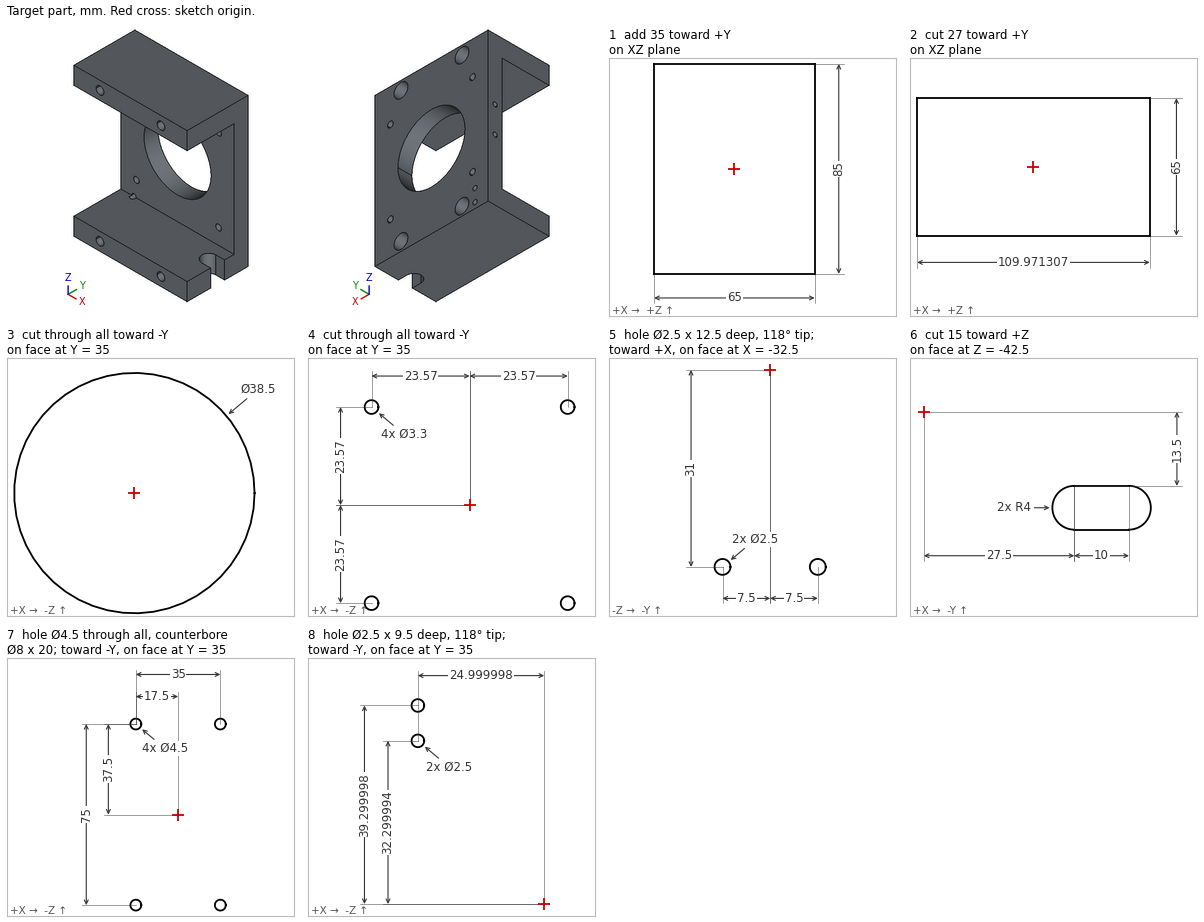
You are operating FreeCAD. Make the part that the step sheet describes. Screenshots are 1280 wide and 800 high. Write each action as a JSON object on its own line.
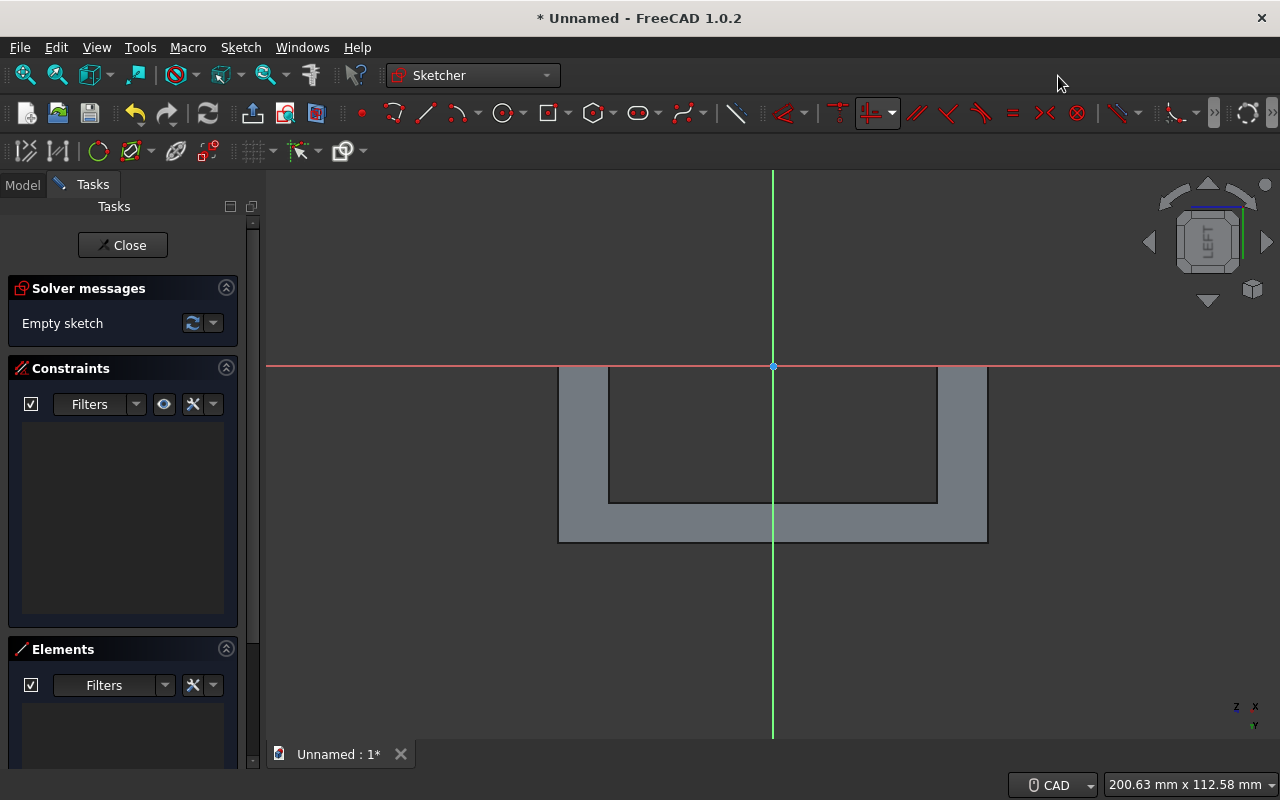
{"action": "scroll", "coordinate": [829, 442], "scroll_direction": "up", "scroll_amount": 4}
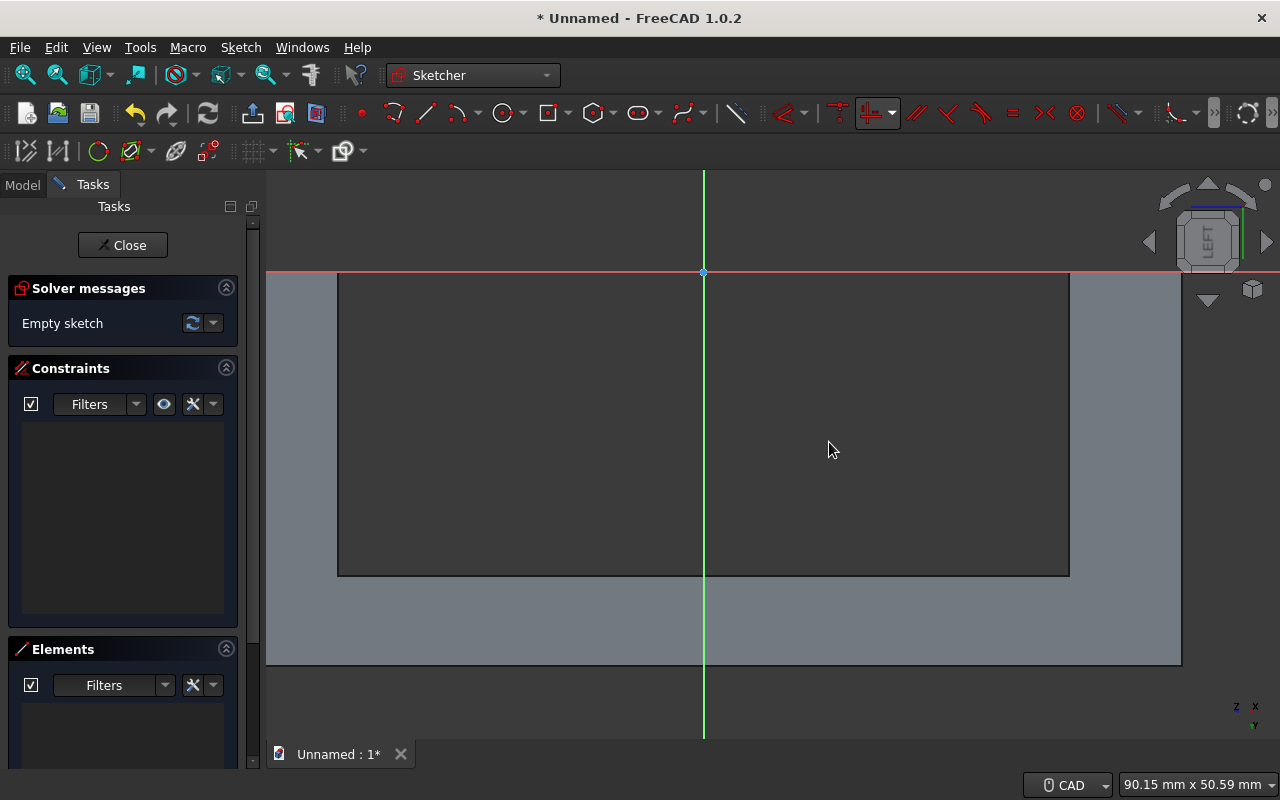
{"action": "left_click", "coordinate": [504, 114]}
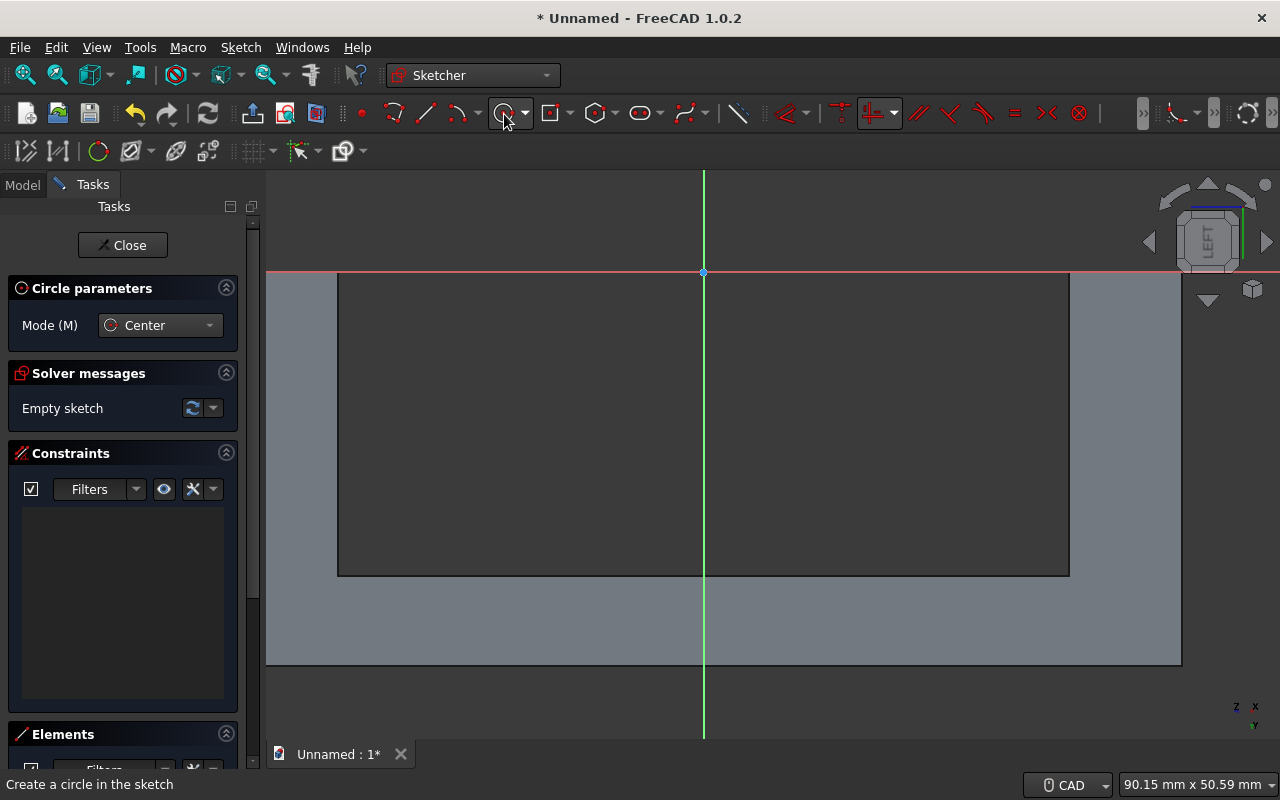
{"action": "scroll", "coordinate": [619, 621], "scroll_direction": "up", "scroll_amount": 3}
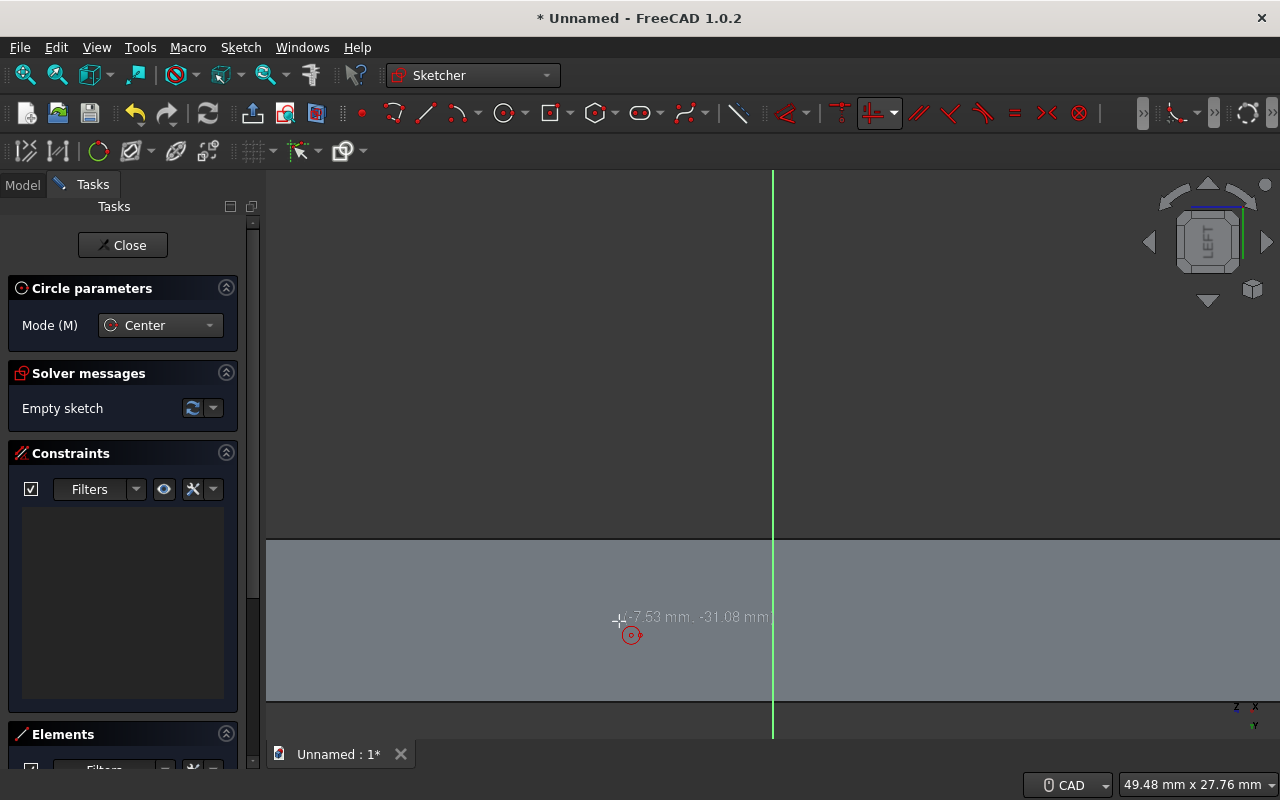
{"action": "left_click", "coordinate": [619, 620]}
{"action": "mouse_move", "coordinate": [637, 602]}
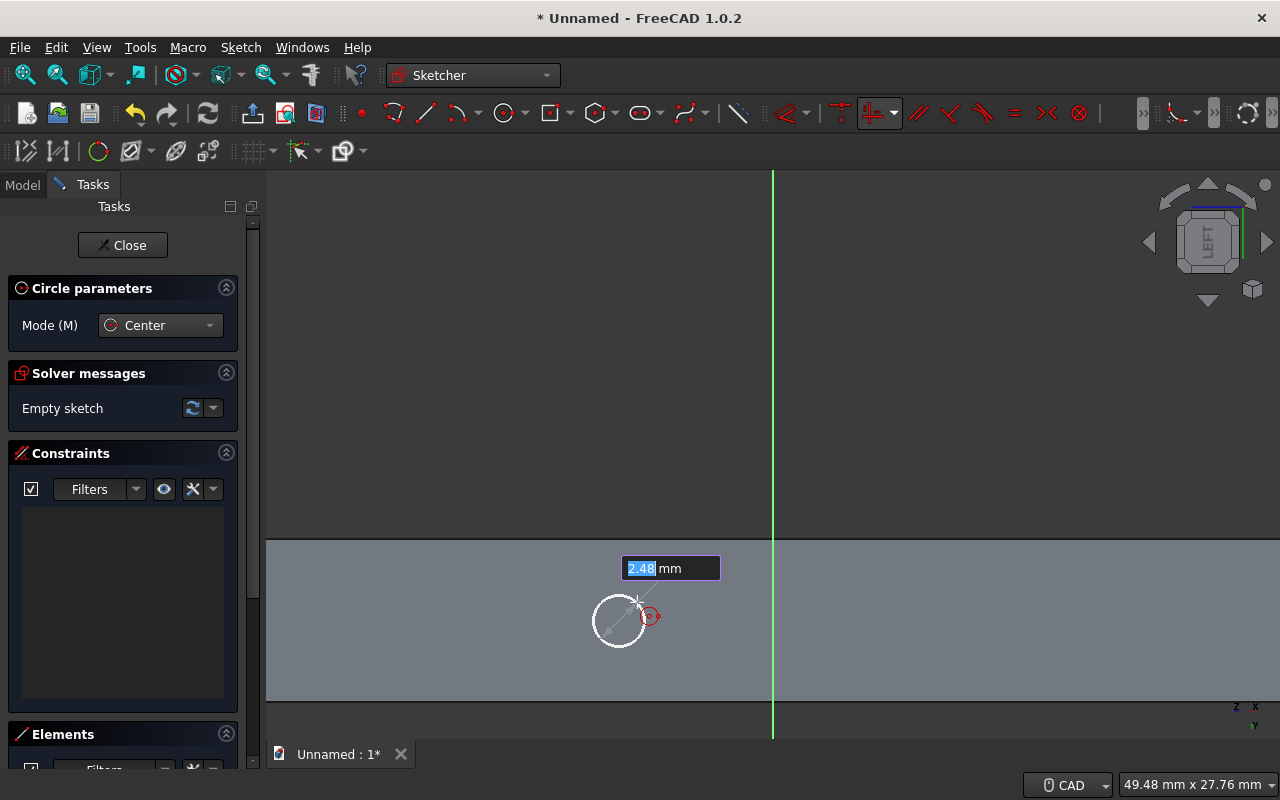
{"action": "type", "text": "2.5"}
{"action": "key", "text": "Return"}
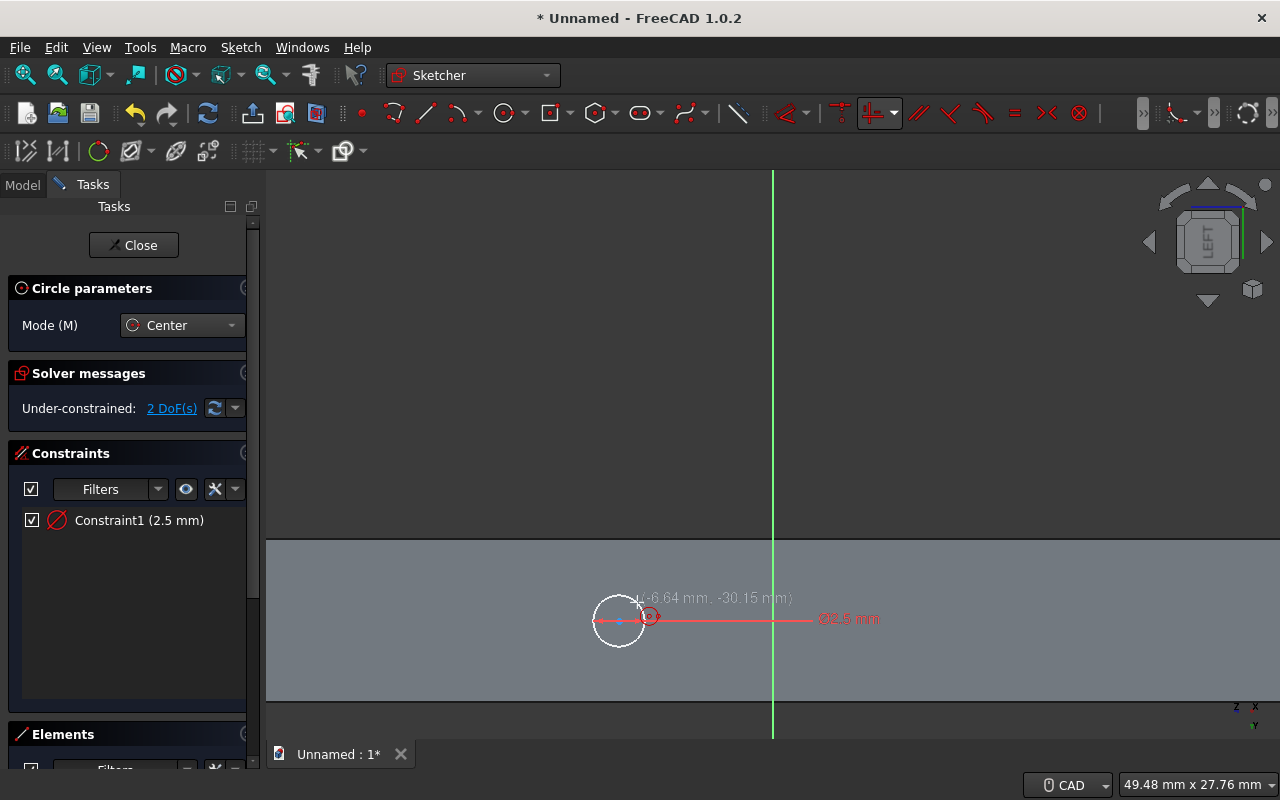
{"action": "left_click", "coordinate": [927, 620]}
{"action": "mouse_move", "coordinate": [945, 602]}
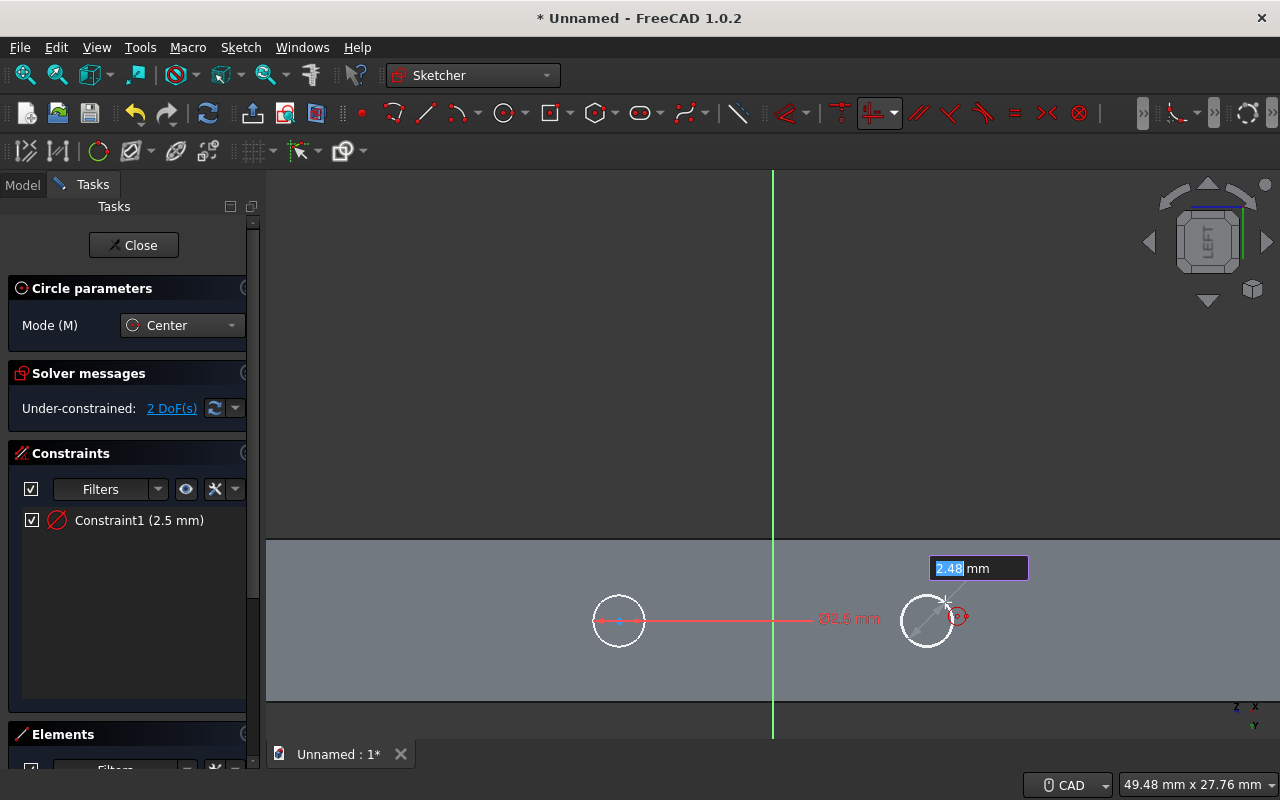
{"action": "type", "text": "2.5"}
{"action": "key", "text": "Return"}
{"action": "key", "text": "Escape"}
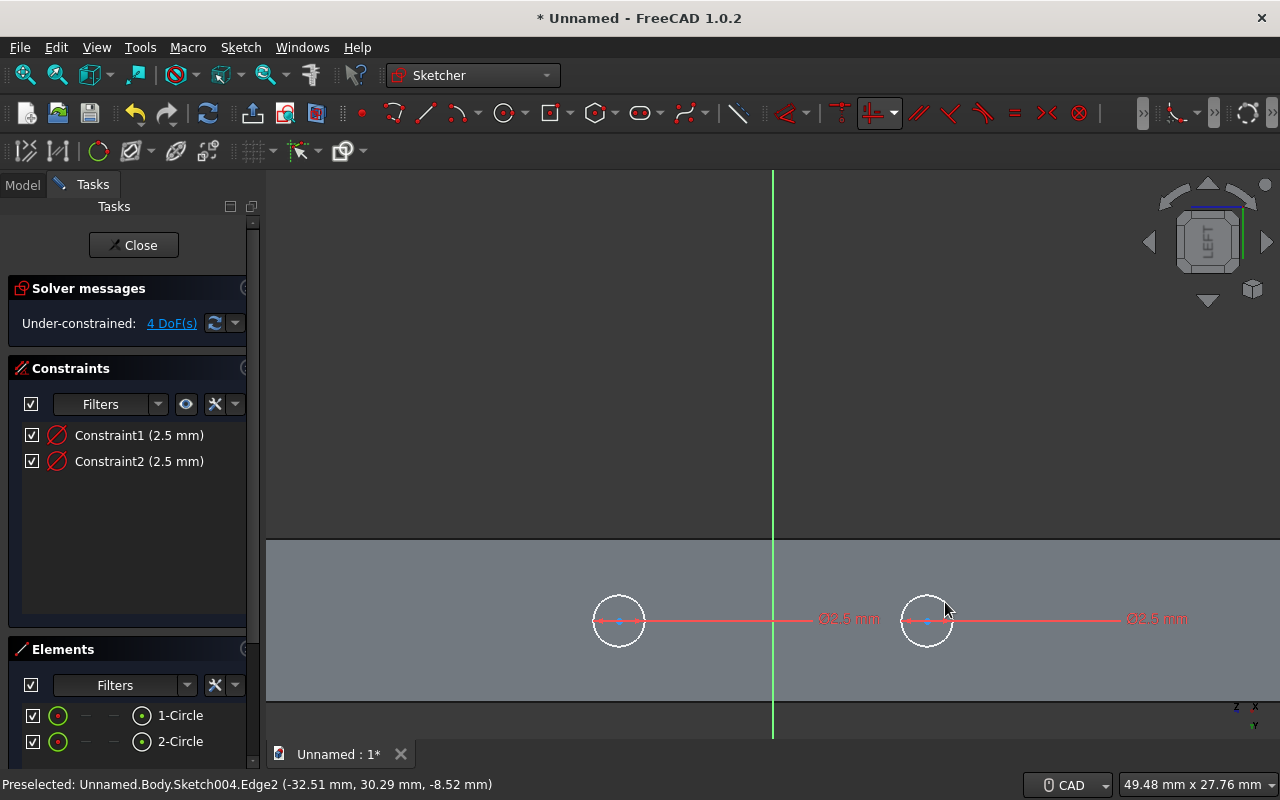
{"action": "left_click", "coordinate": [619, 621]}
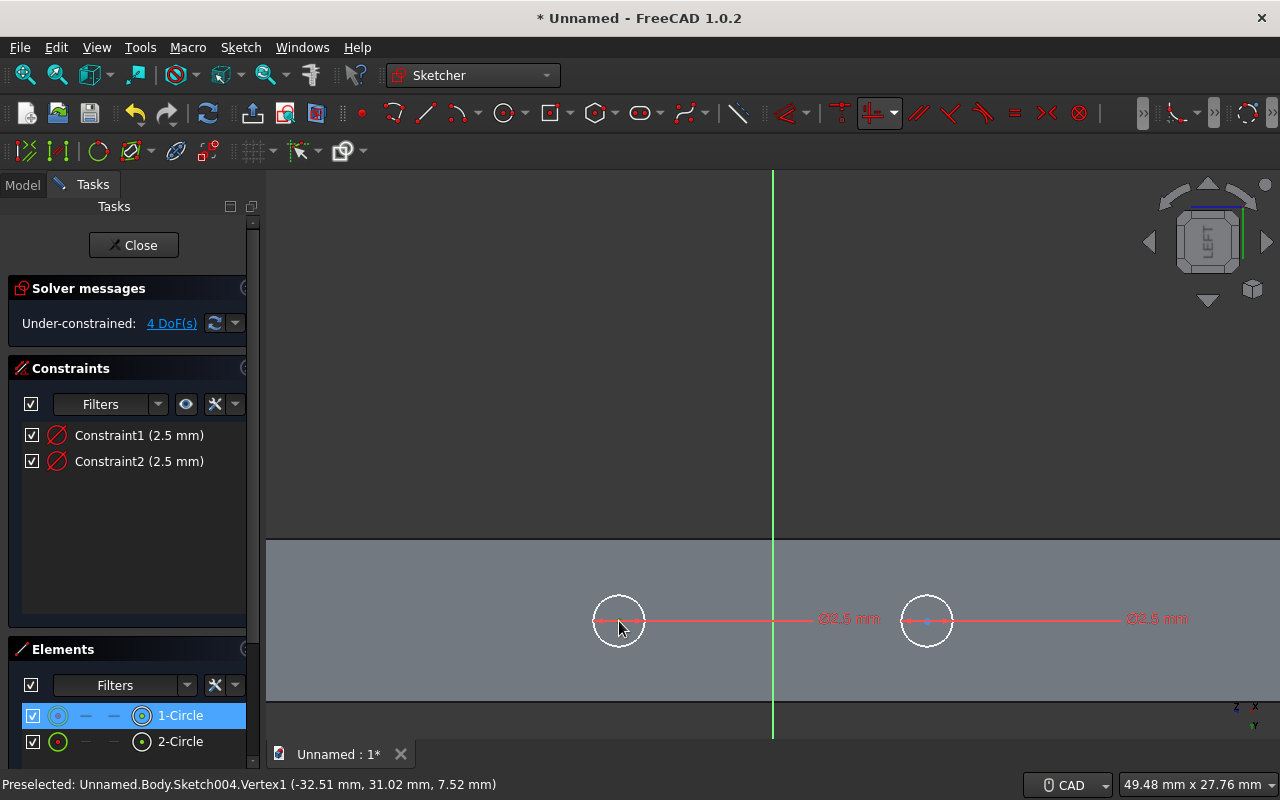
{"action": "left_click", "coordinate": [927, 621]}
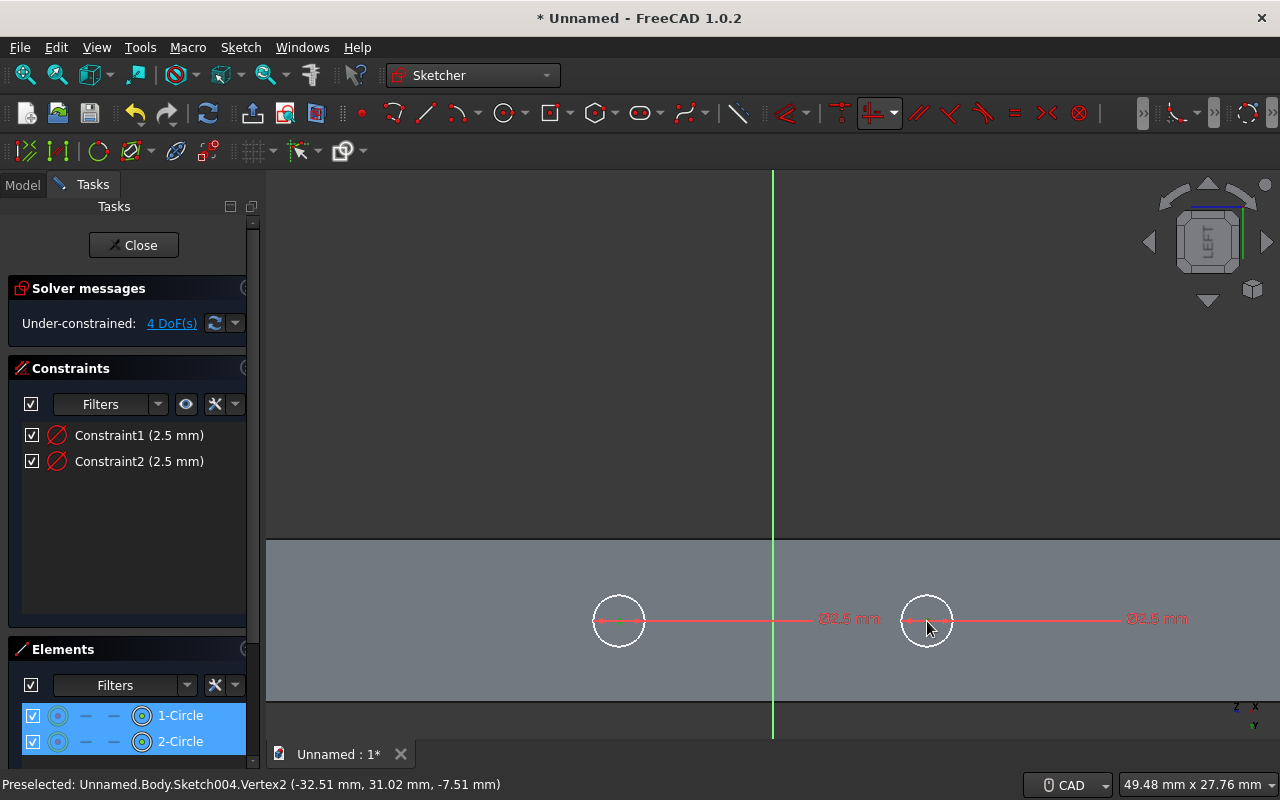
{"action": "key", "text": "h"}